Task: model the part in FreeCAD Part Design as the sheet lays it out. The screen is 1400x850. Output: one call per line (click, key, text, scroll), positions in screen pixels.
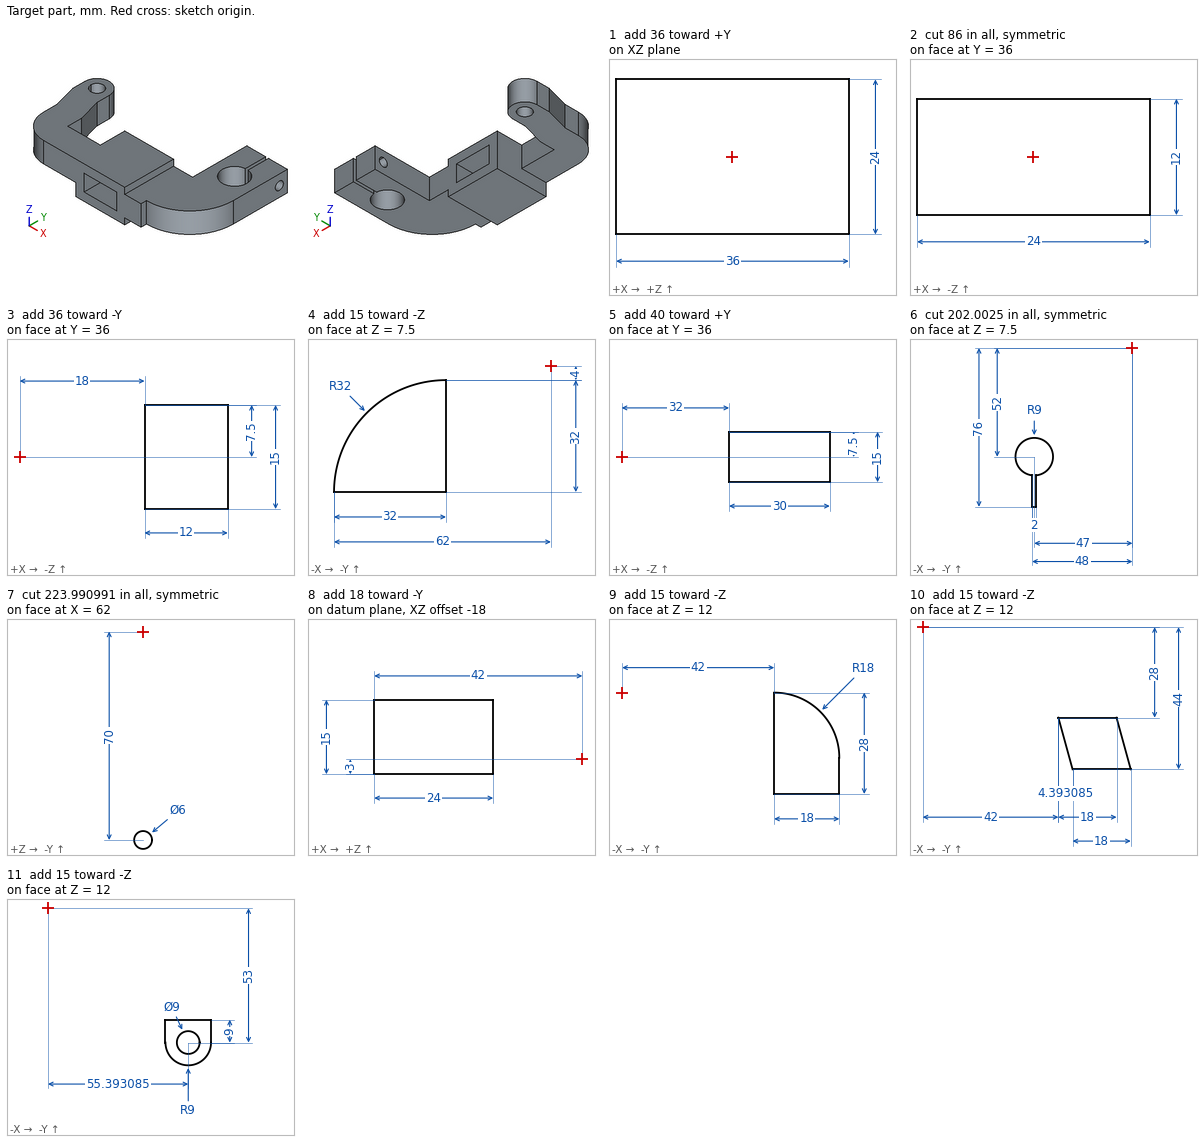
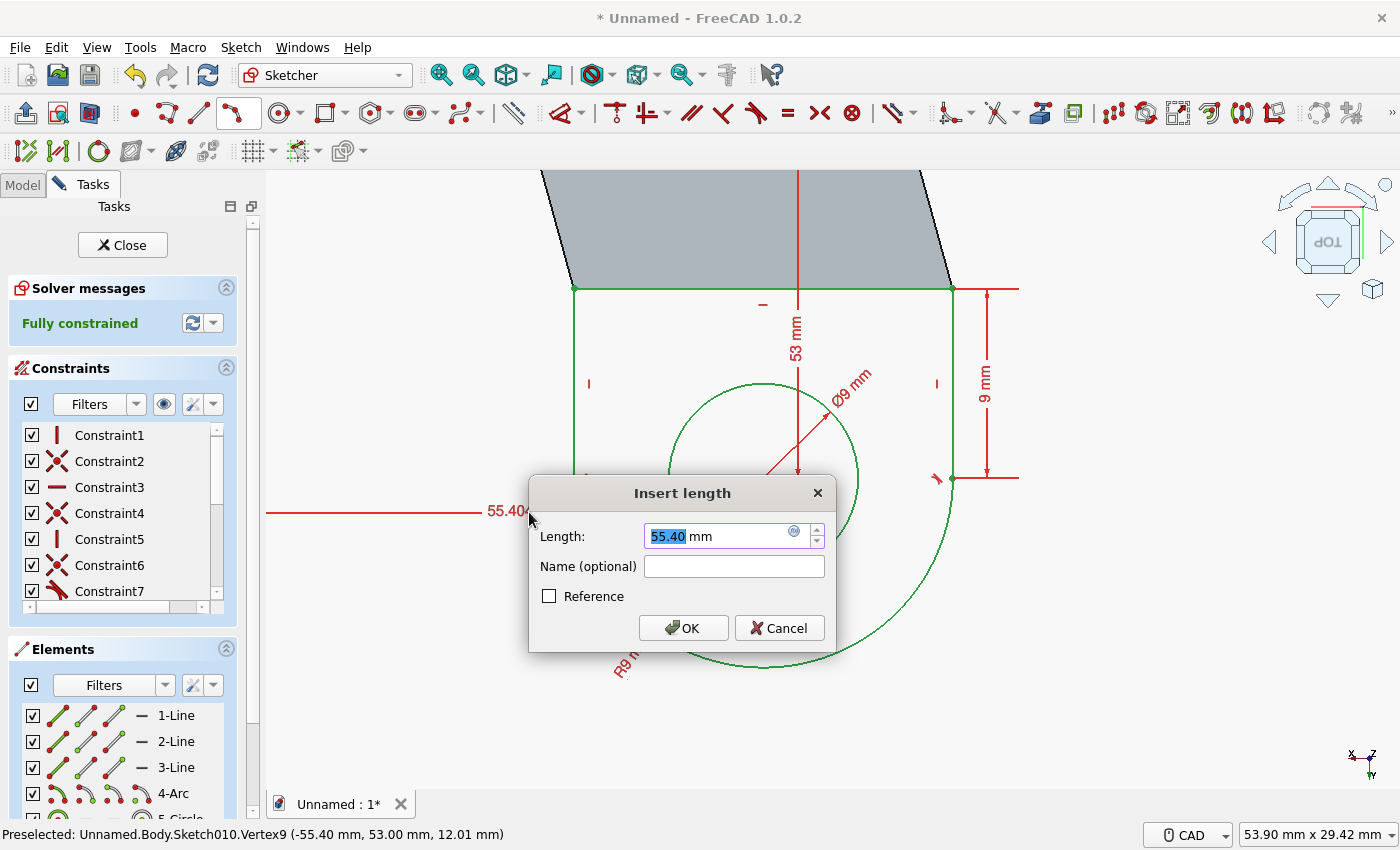
text(55.393085)
key(Return)
key(Escape)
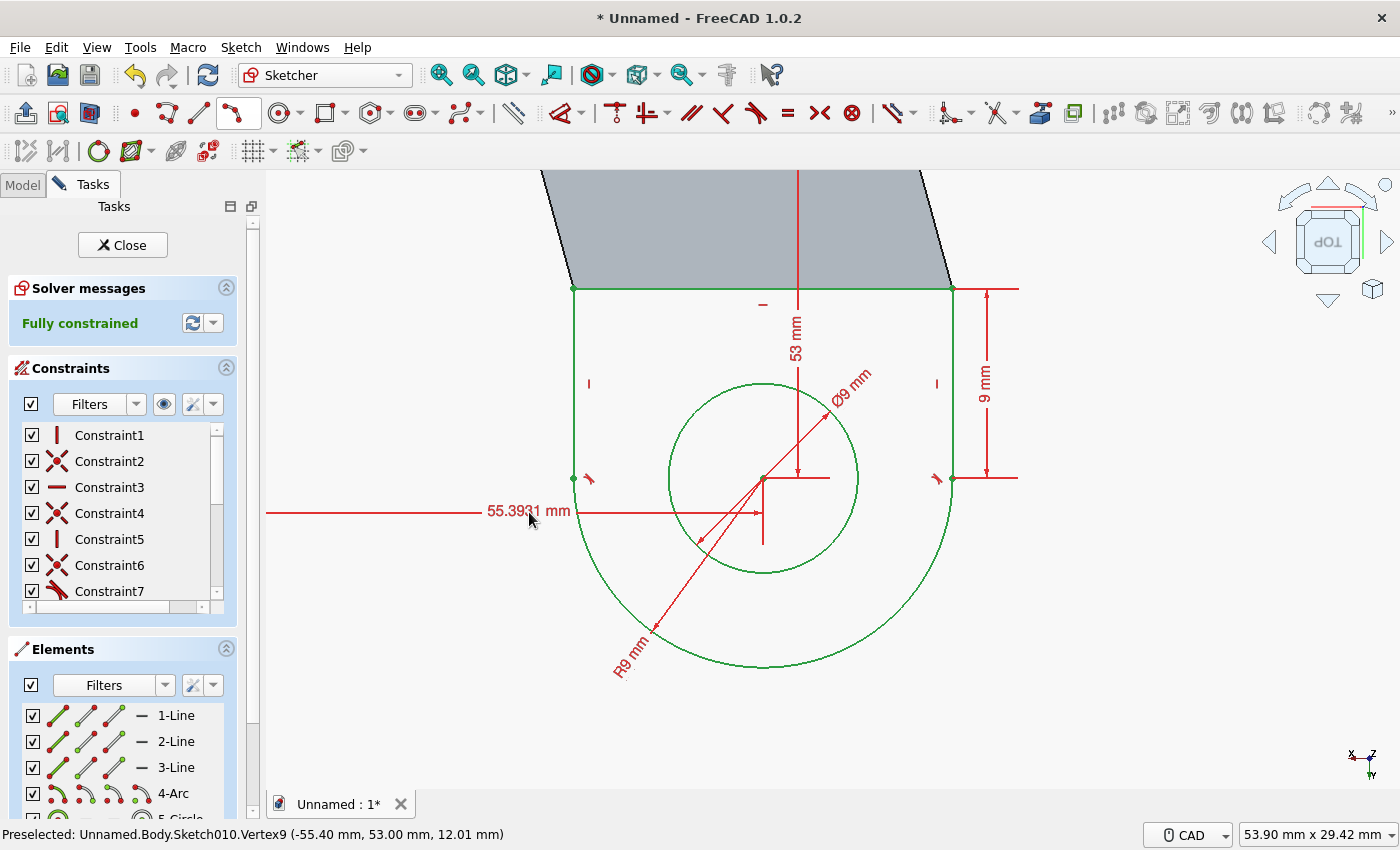
click(123, 245)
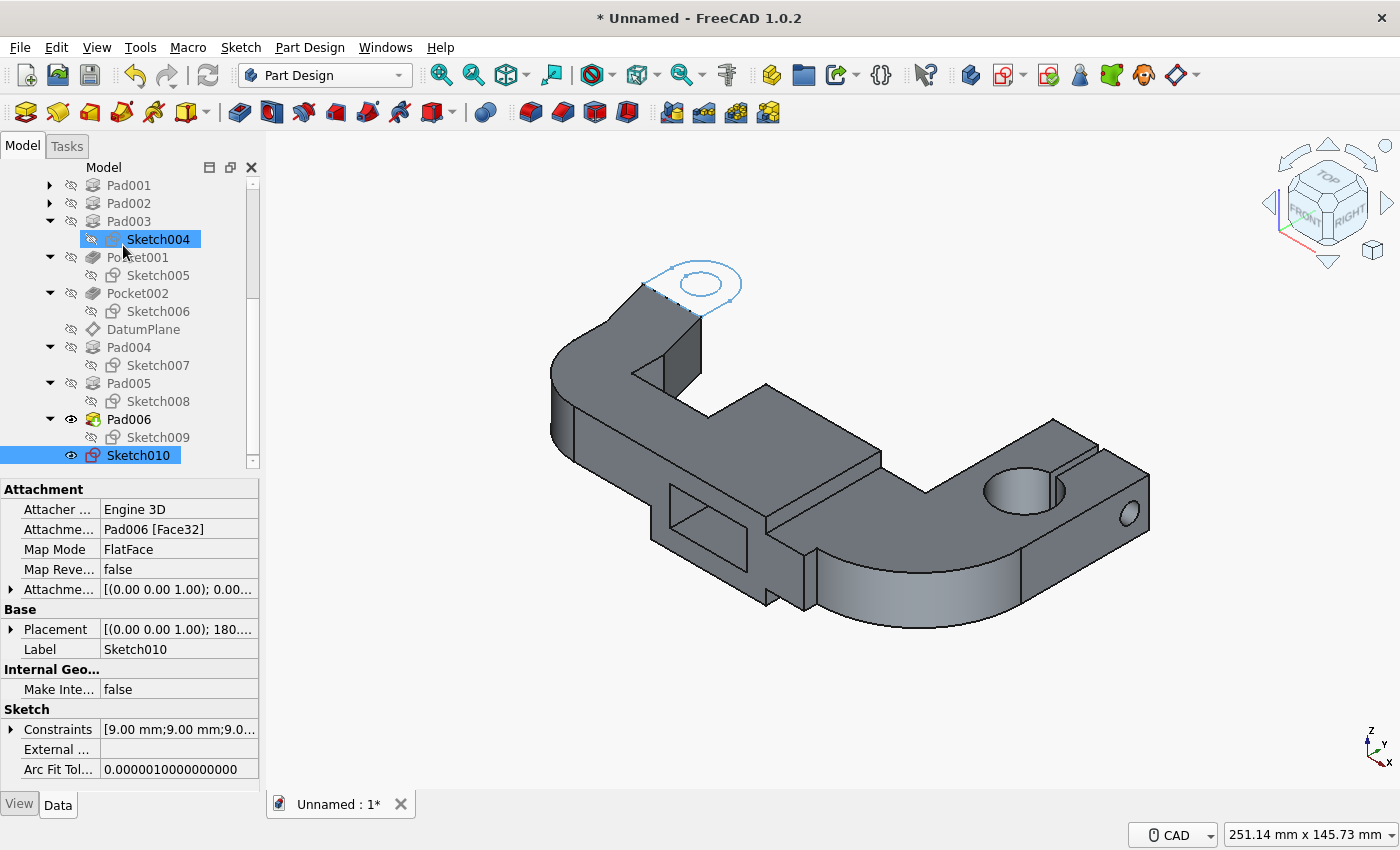
click(26, 112)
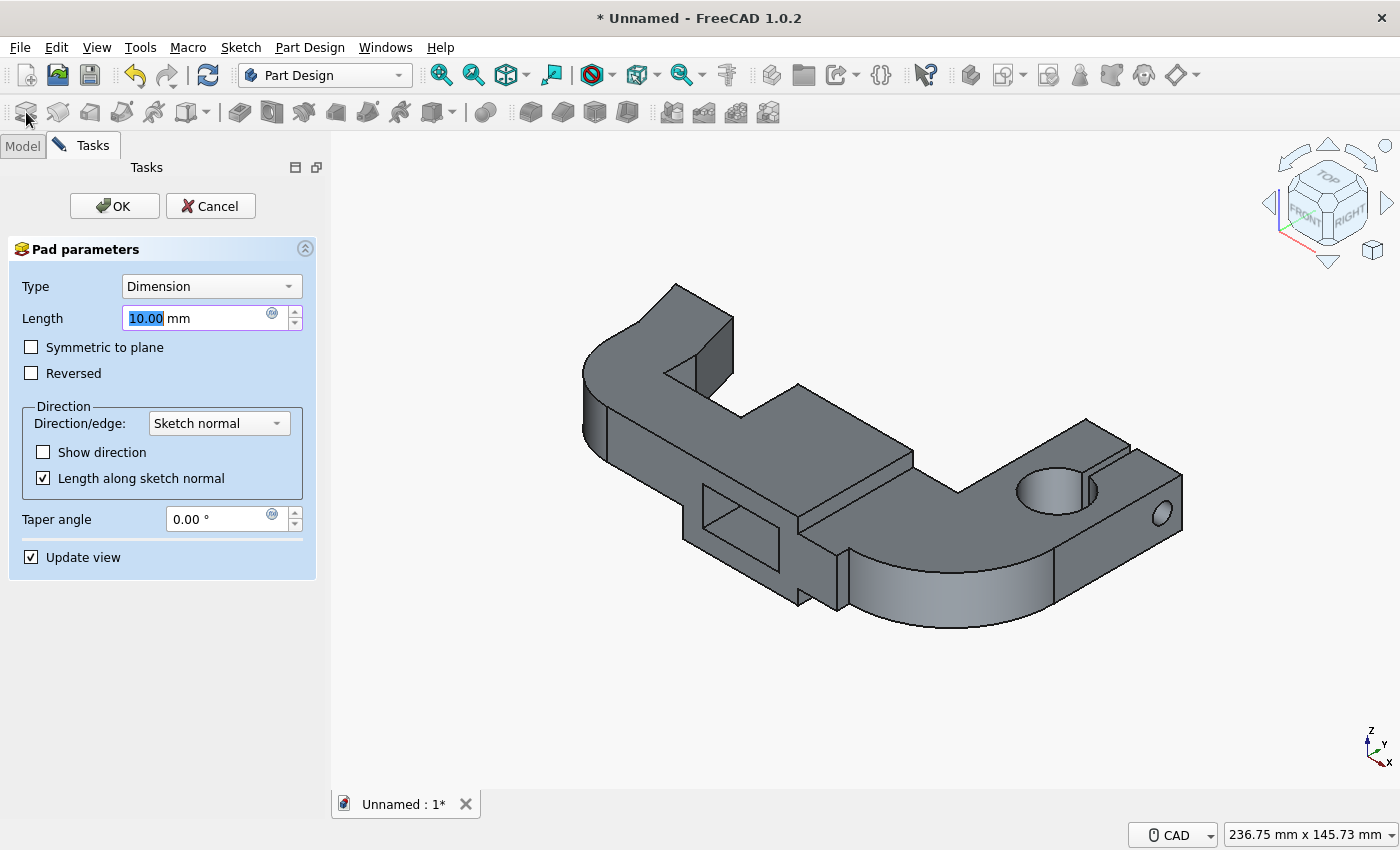
text(15)
key(Tab)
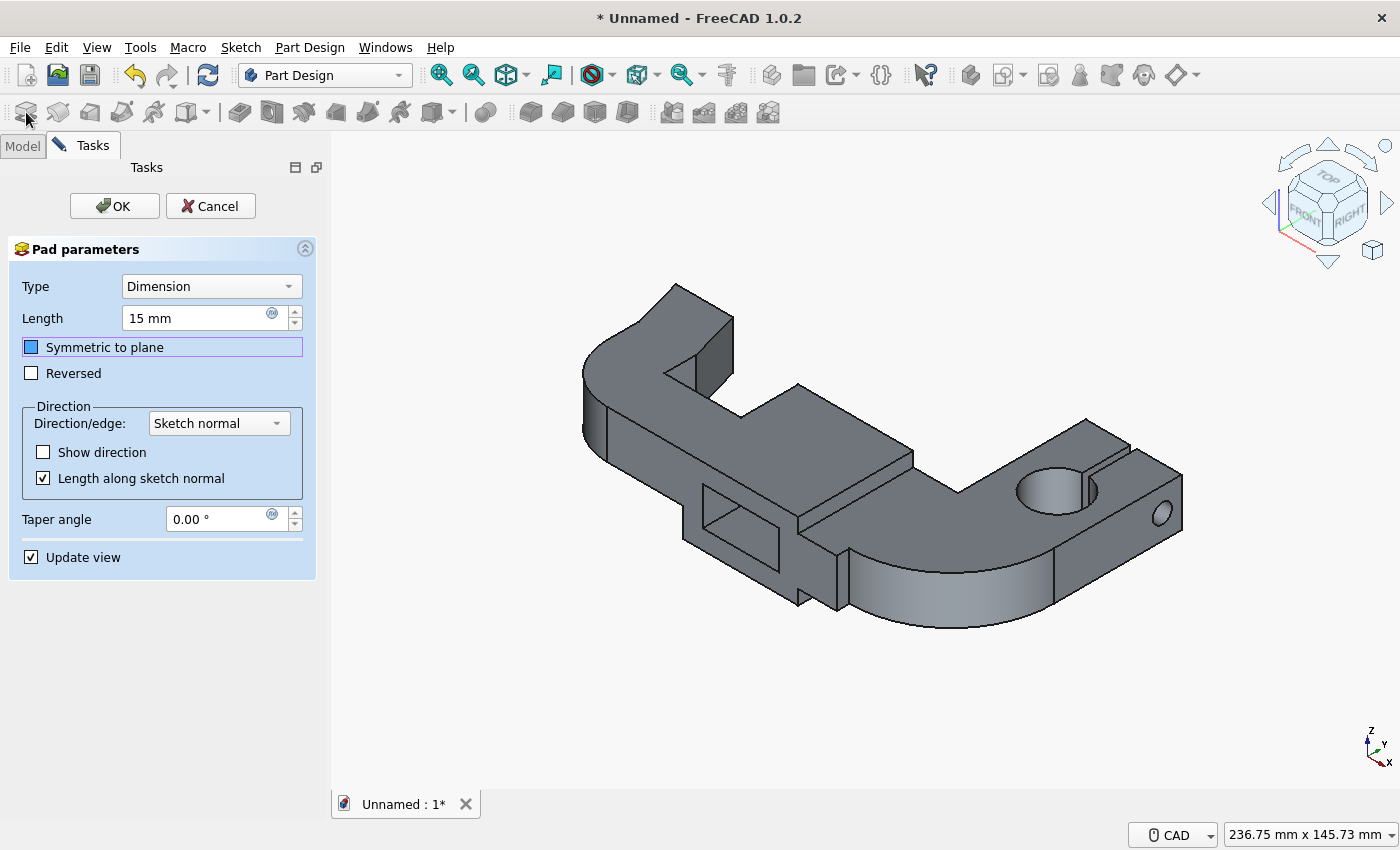
click(30, 373)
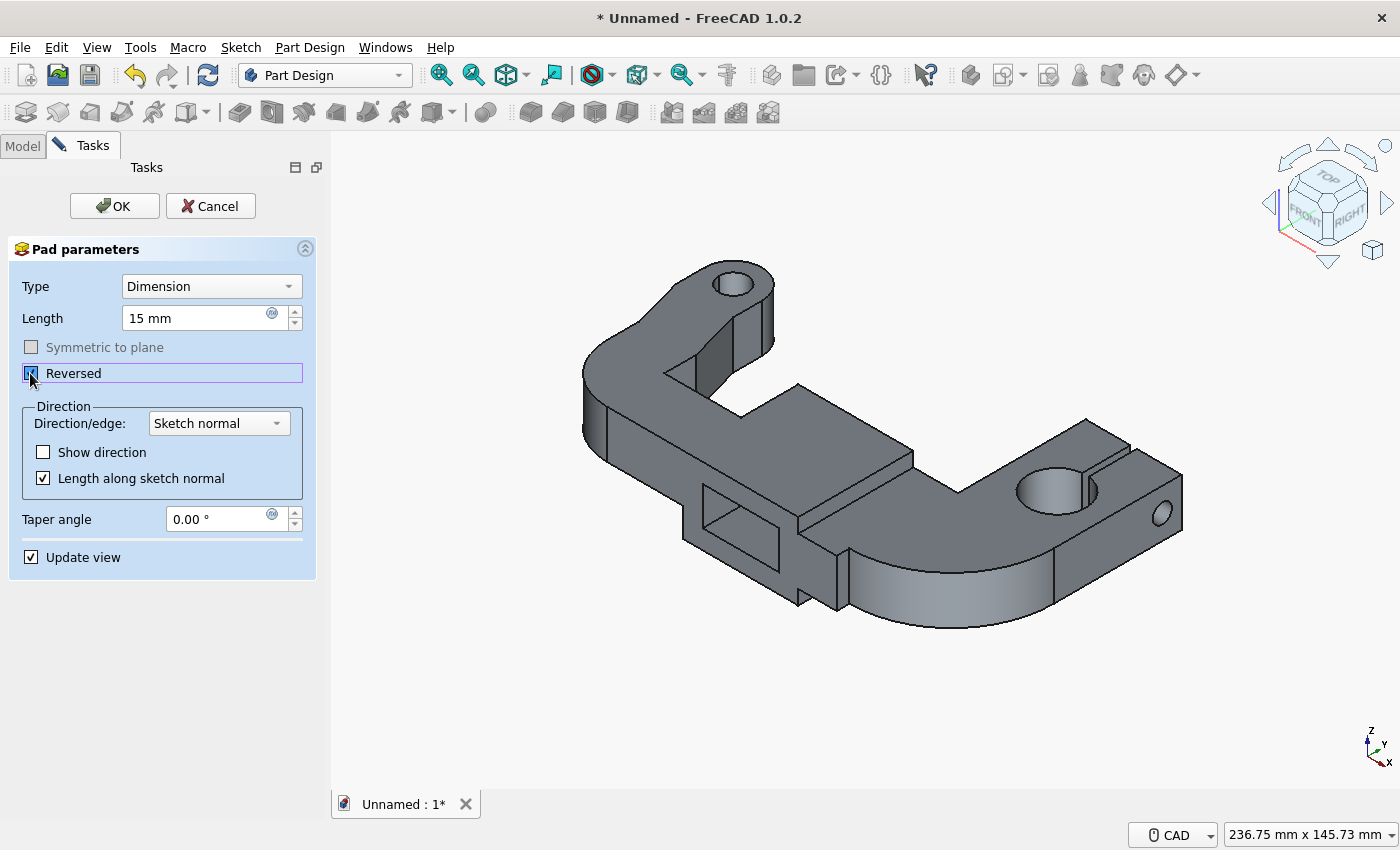
click(115, 206)